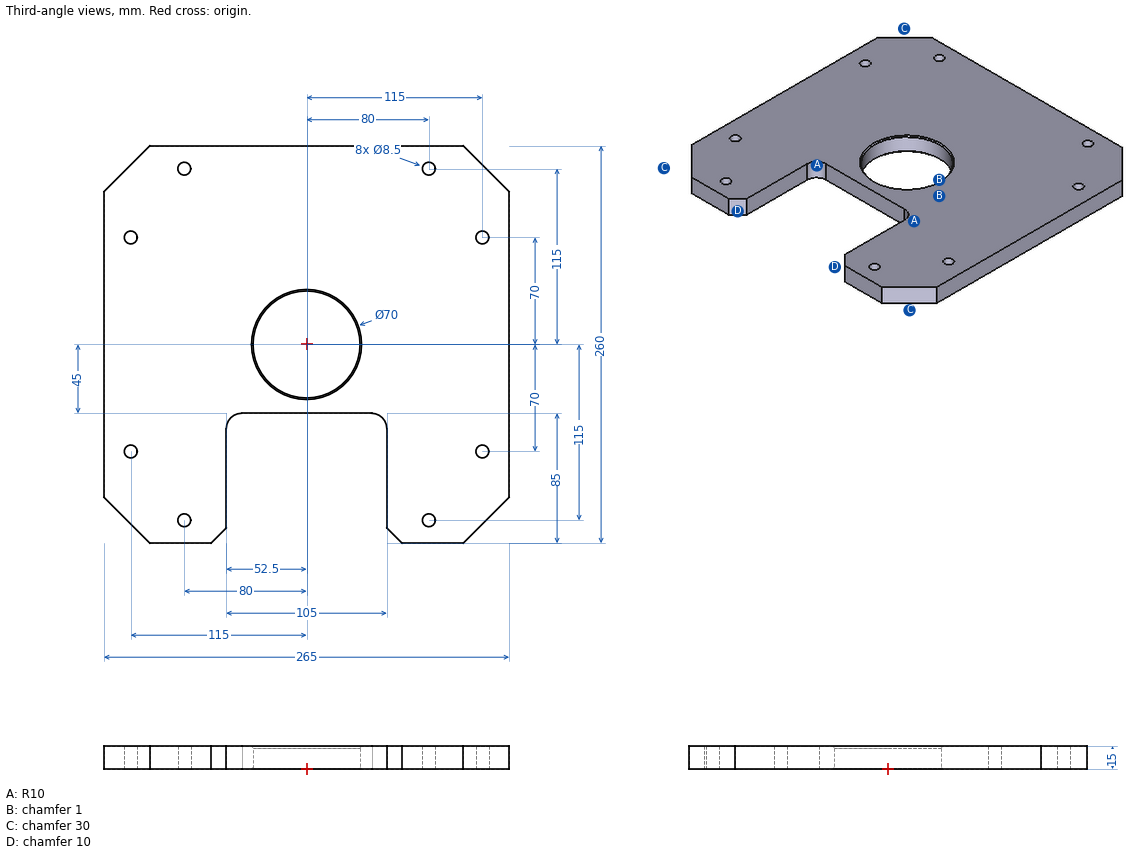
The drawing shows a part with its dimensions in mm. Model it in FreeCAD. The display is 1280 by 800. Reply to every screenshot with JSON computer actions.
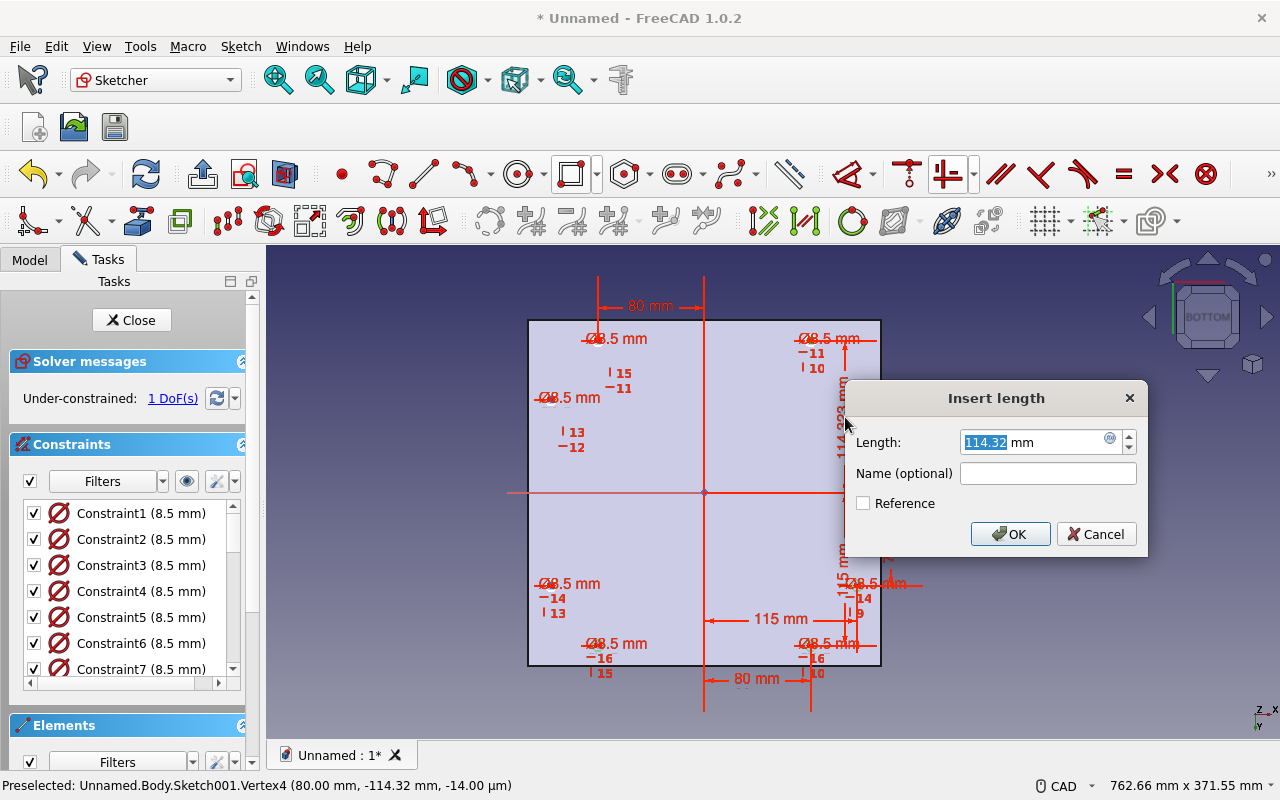
{"action": "type", "text": "115"}
{"action": "key", "text": "Return"}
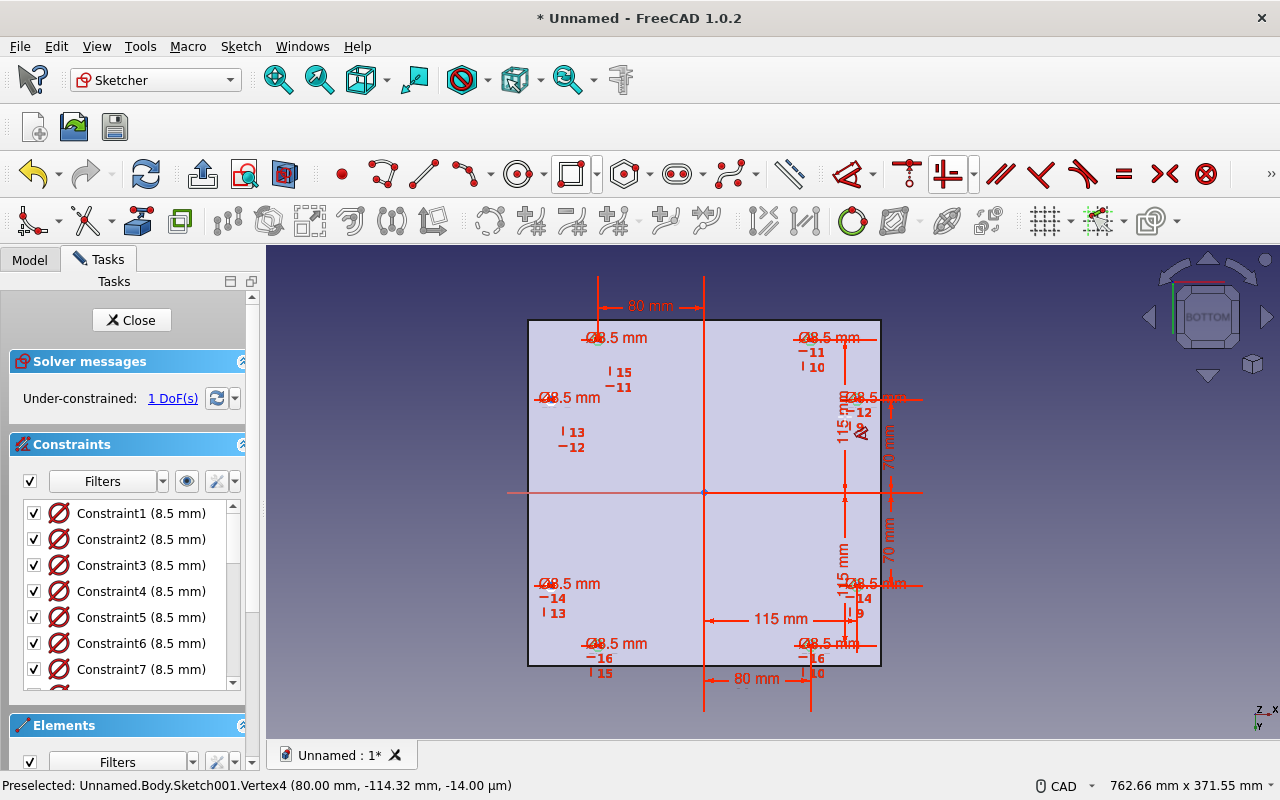
{"action": "left_click", "coordinate": [551, 400]}
{"action": "left_click", "coordinate": [628, 366]}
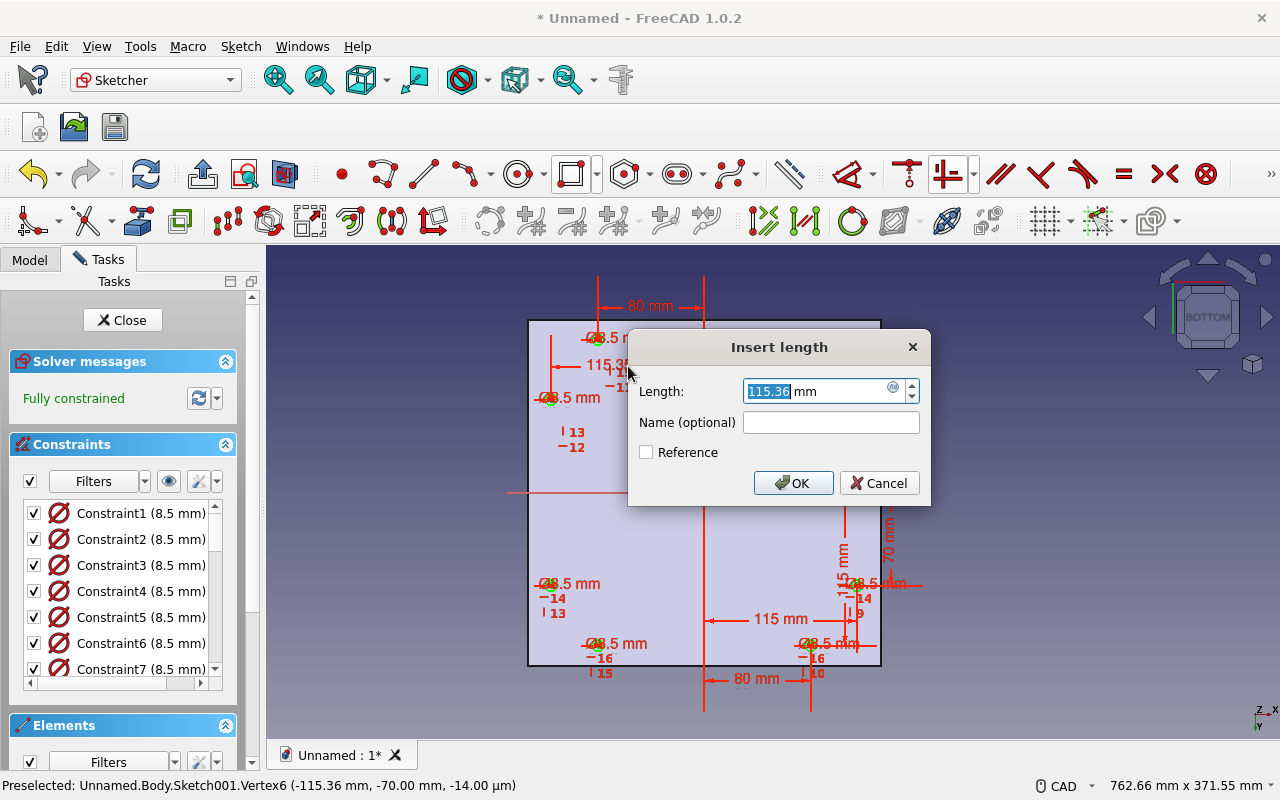
{"action": "type", "text": "115"}
{"action": "key", "text": "Return"}
{"action": "key", "text": "Escape"}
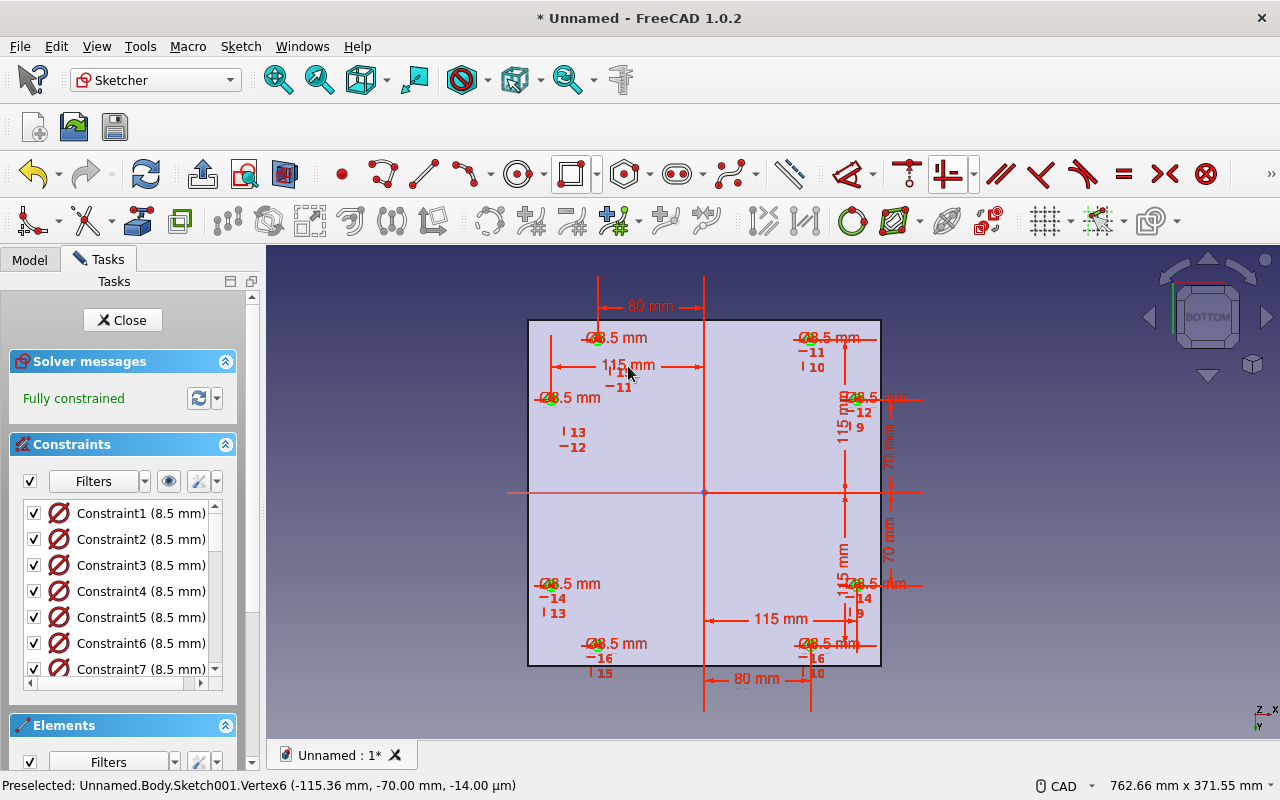
{"action": "left_click", "coordinate": [123, 320]}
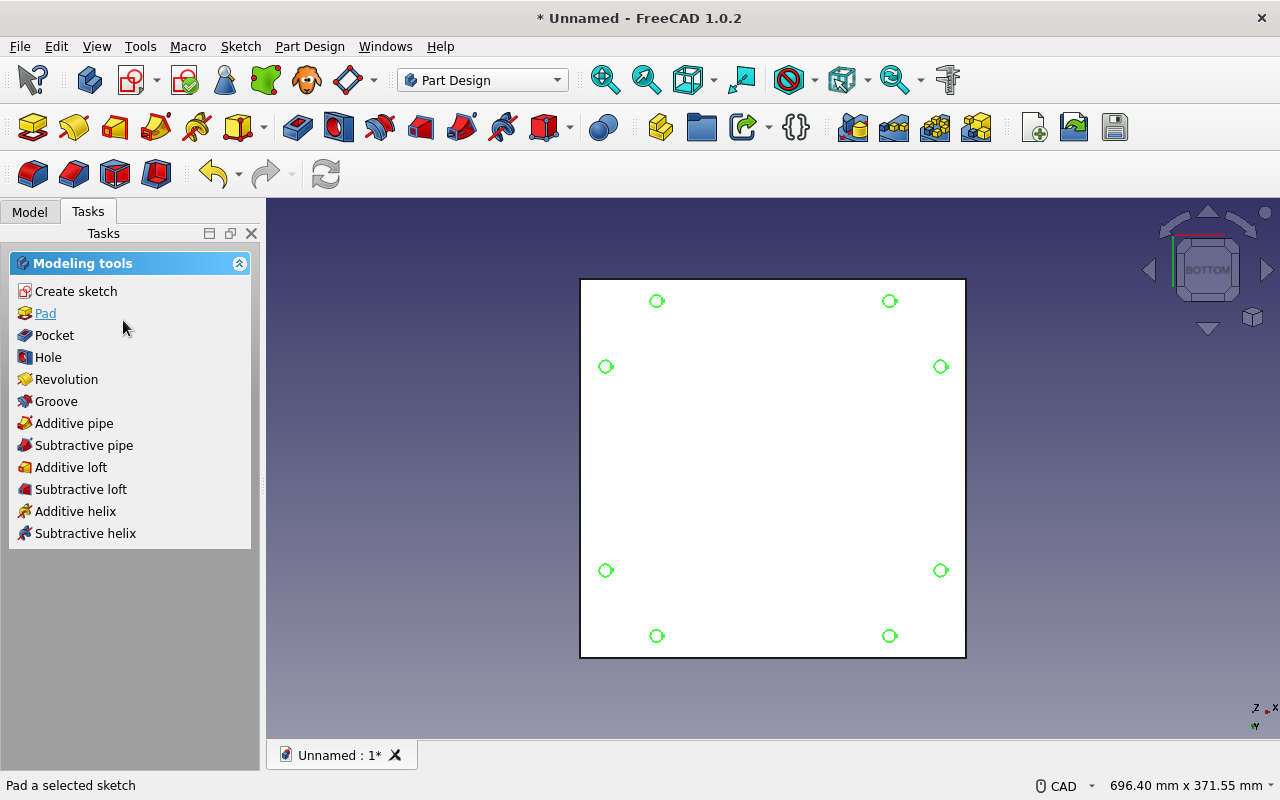
{"action": "left_click", "coordinate": [298, 128]}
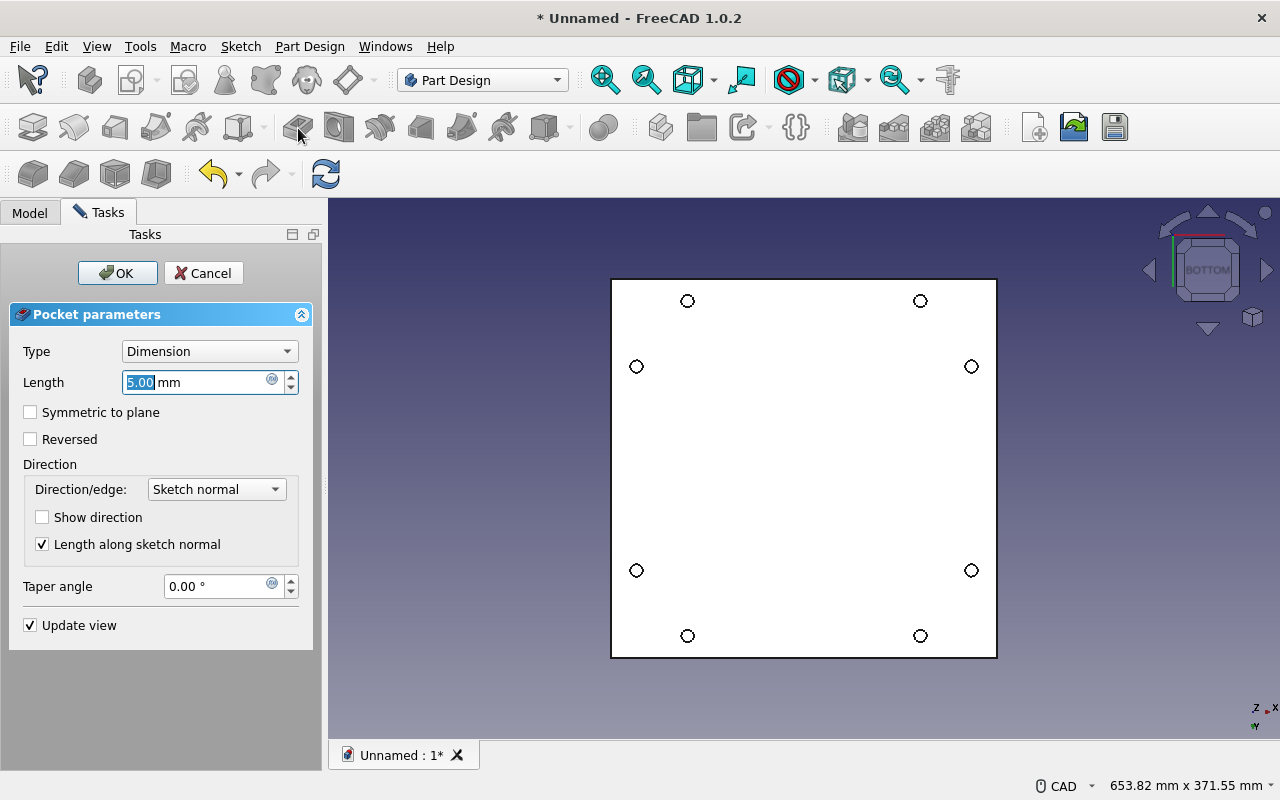
{"action": "left_click", "coordinate": [210, 352]}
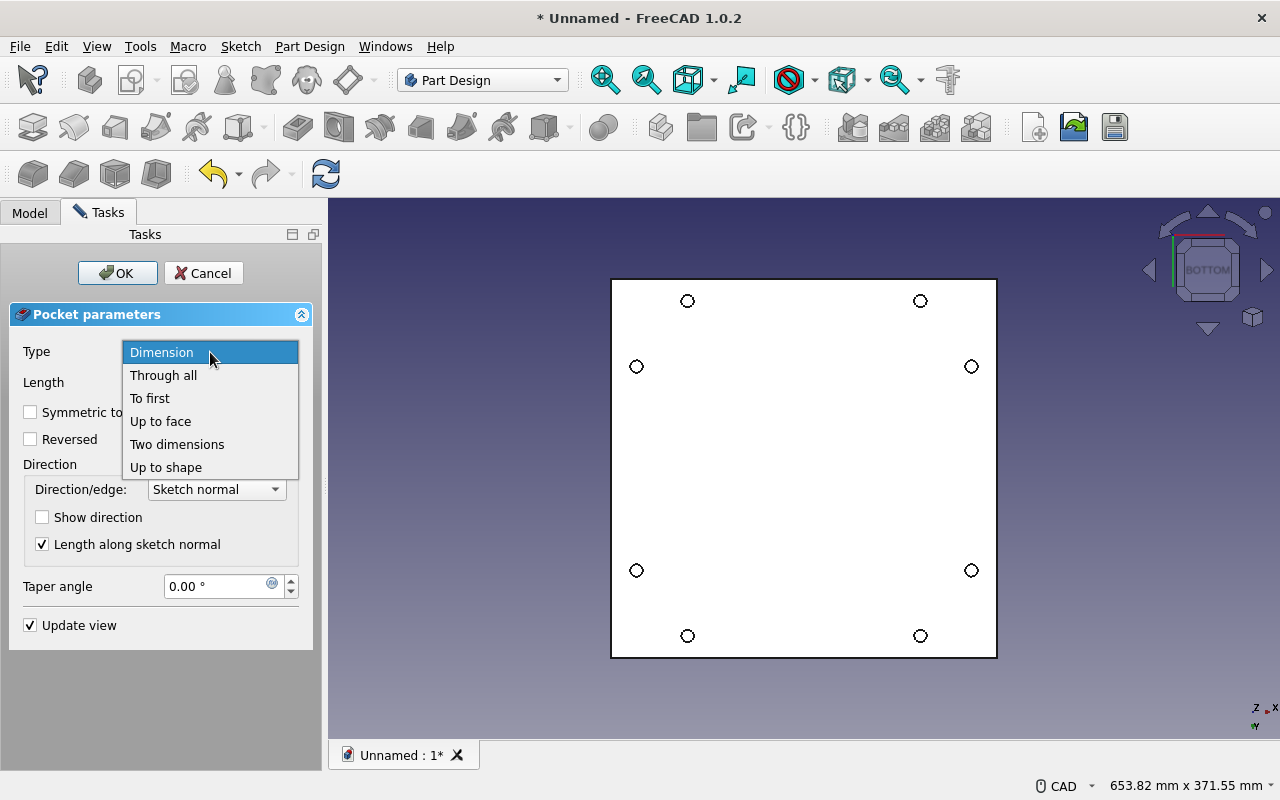
{"action": "left_click", "coordinate": [208, 376]}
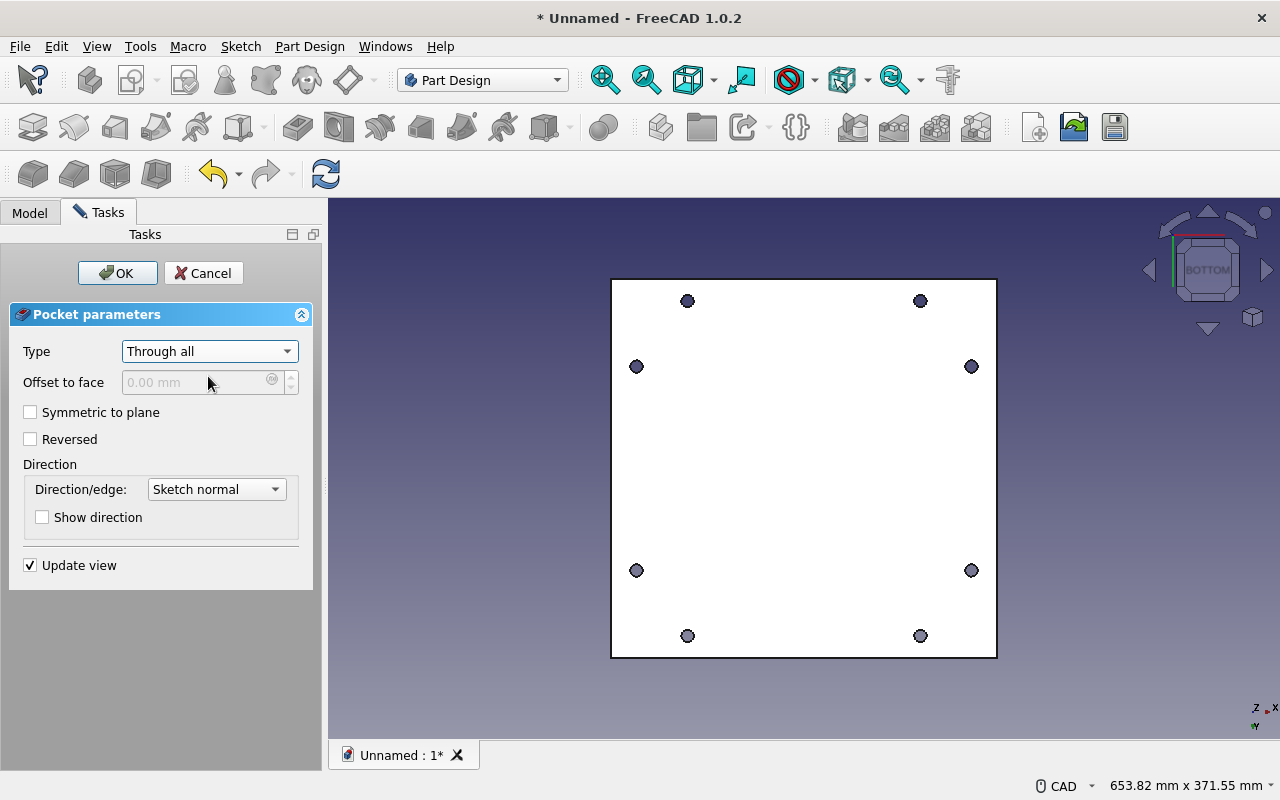
{"action": "left_click", "coordinate": [118, 273]}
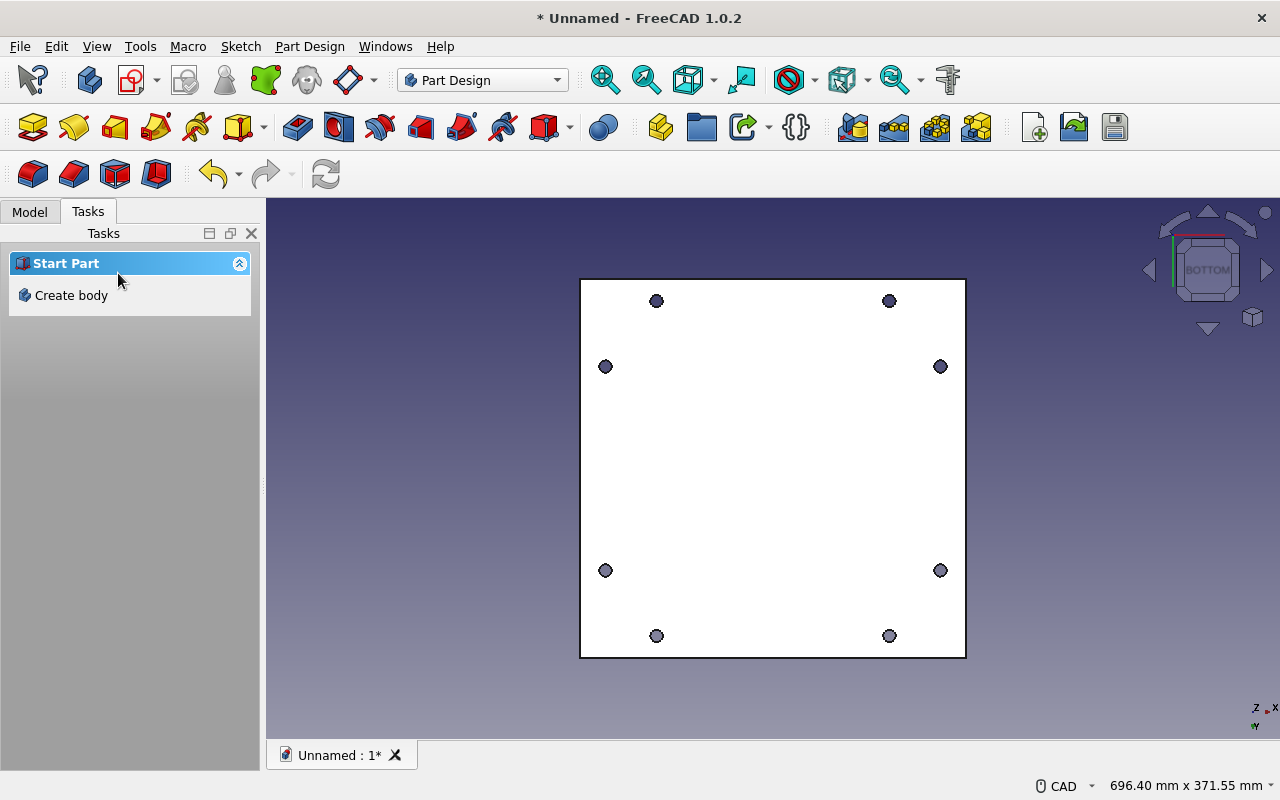
{"action": "left_click", "coordinate": [773, 468]}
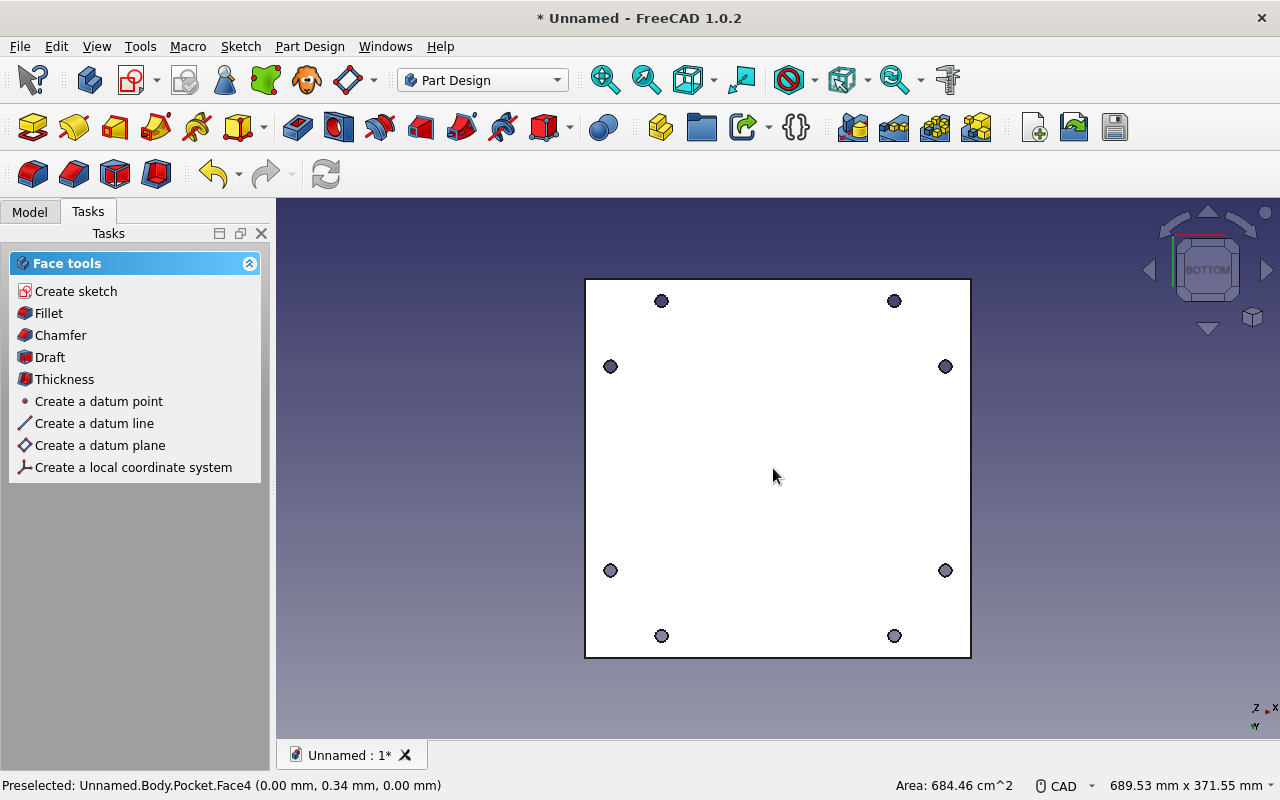
{"action": "left_click", "coordinate": [130, 80]}